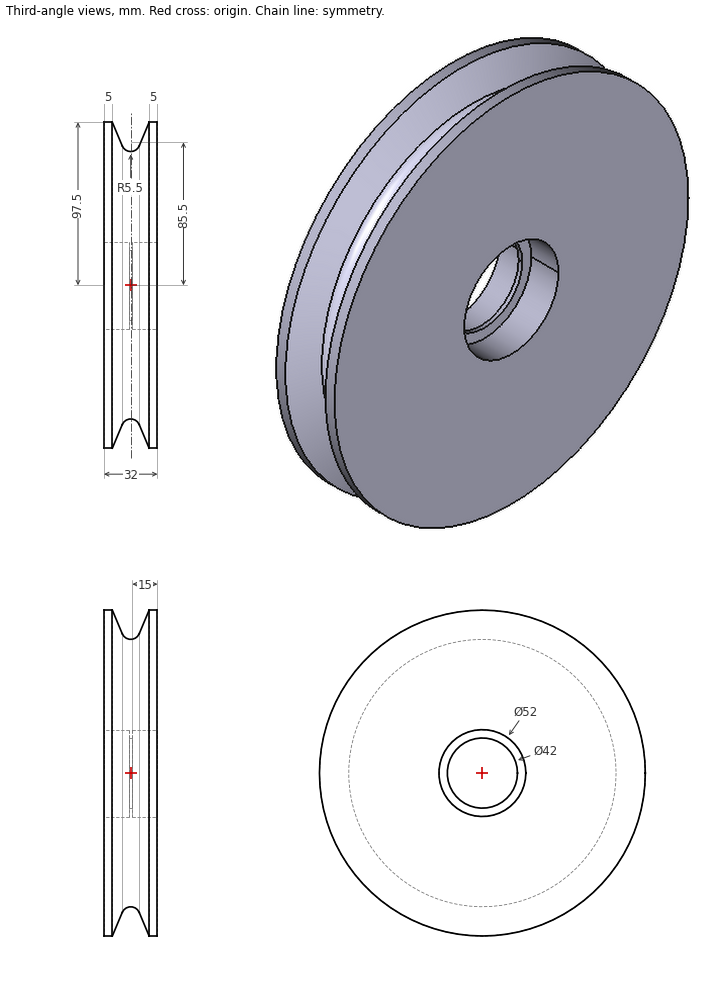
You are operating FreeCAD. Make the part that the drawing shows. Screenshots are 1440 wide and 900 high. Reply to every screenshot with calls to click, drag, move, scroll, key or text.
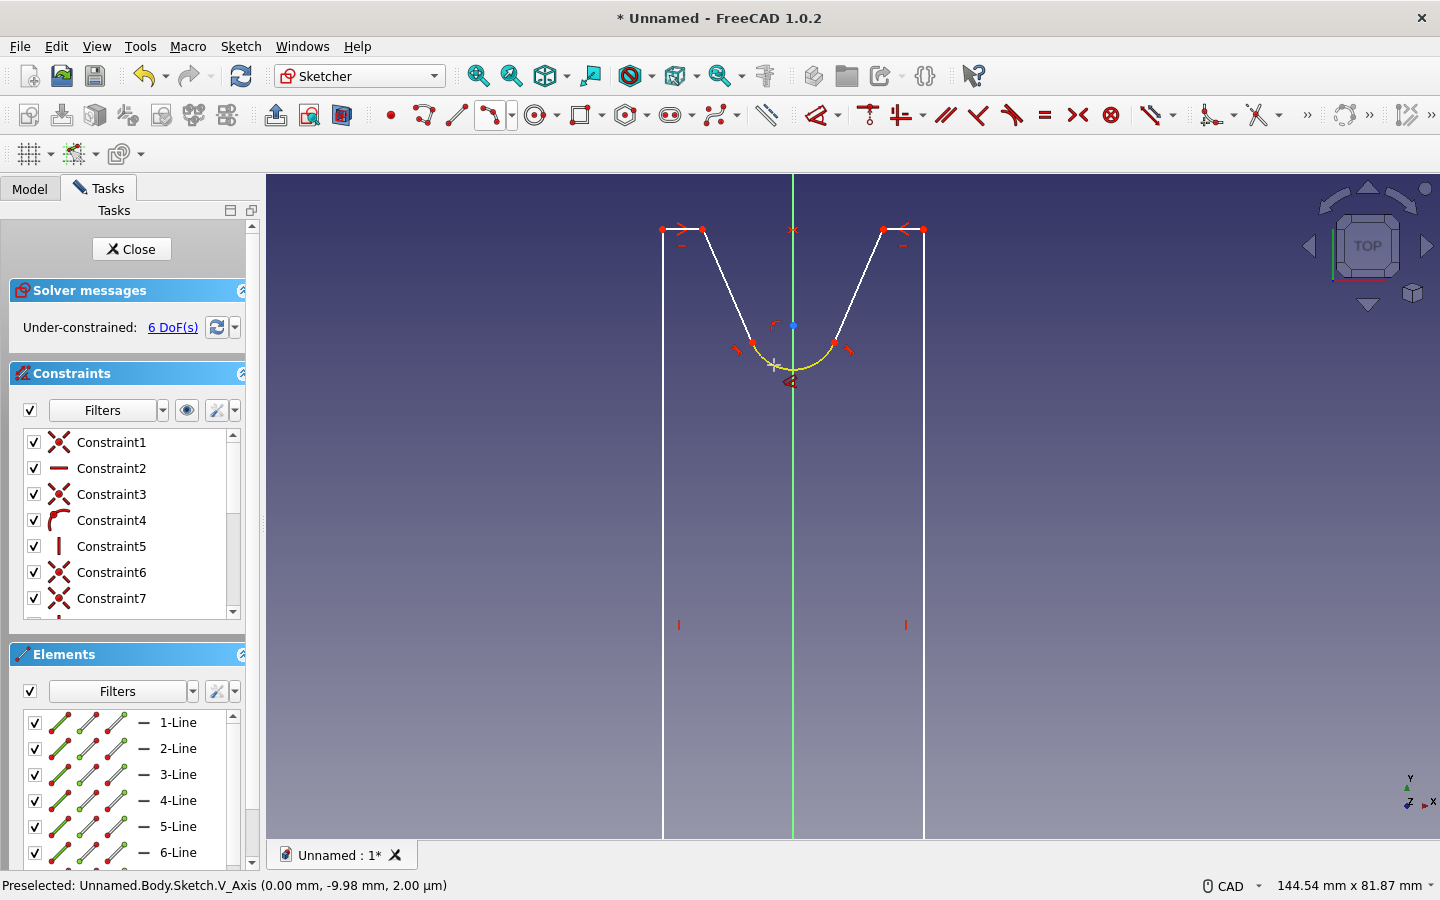
click(773, 365)
click(759, 394)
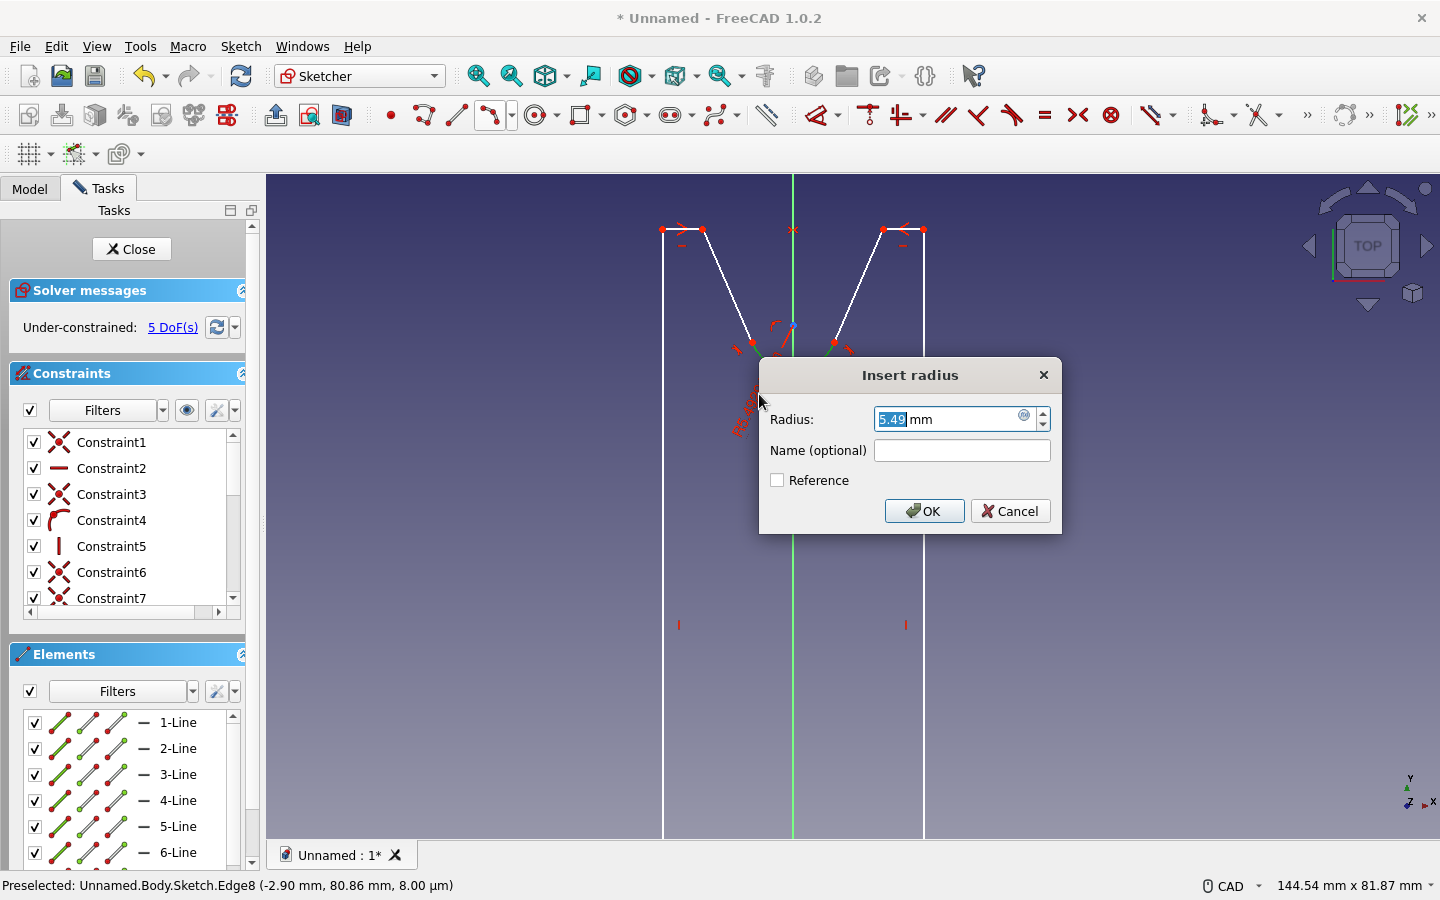
text(5.5)
key(Return)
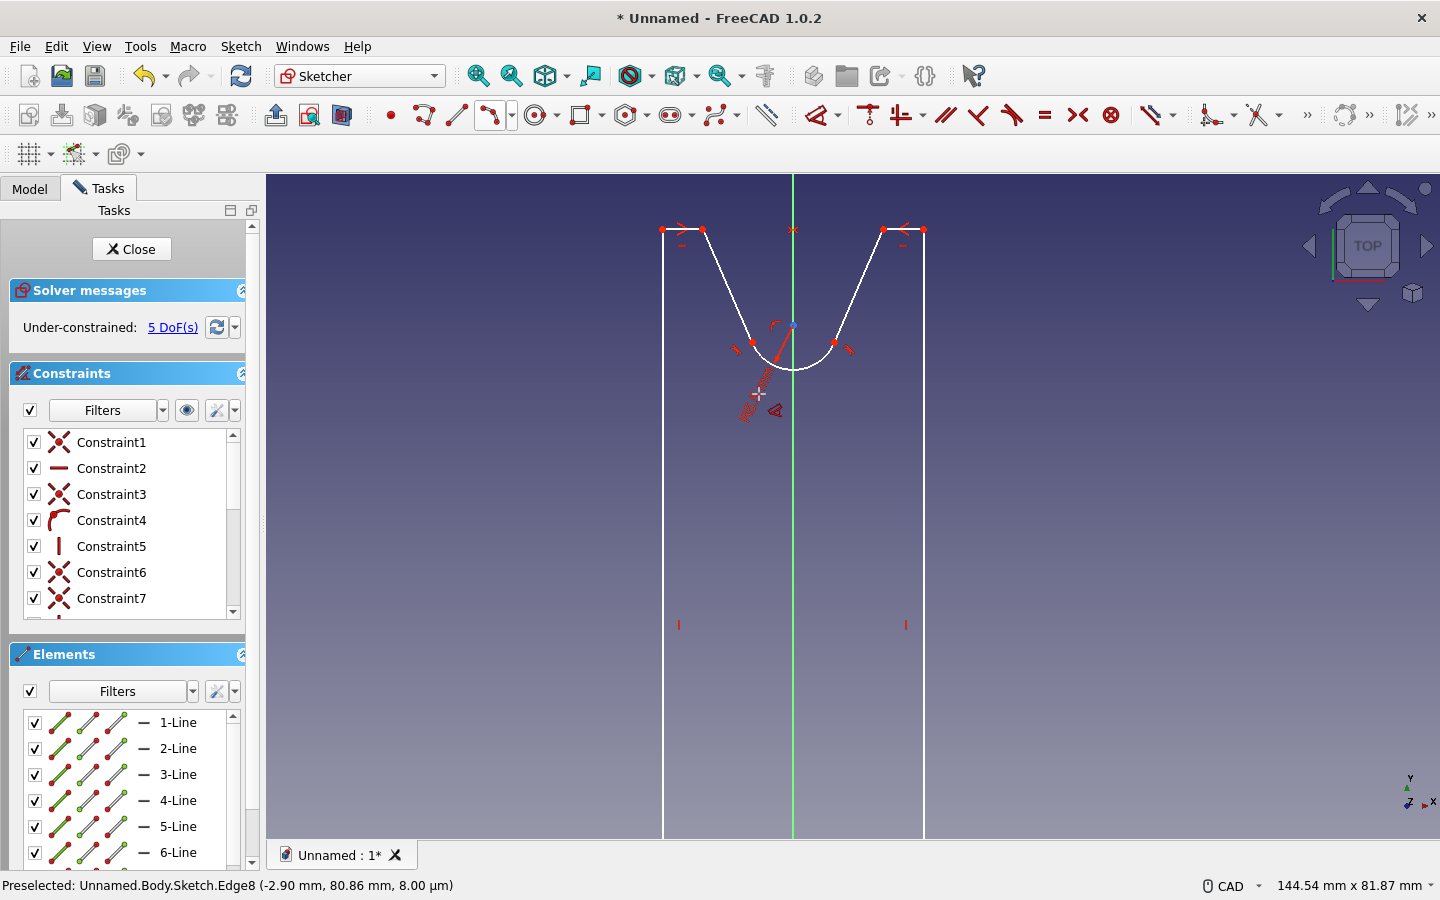
click(691, 229)
click(683, 263)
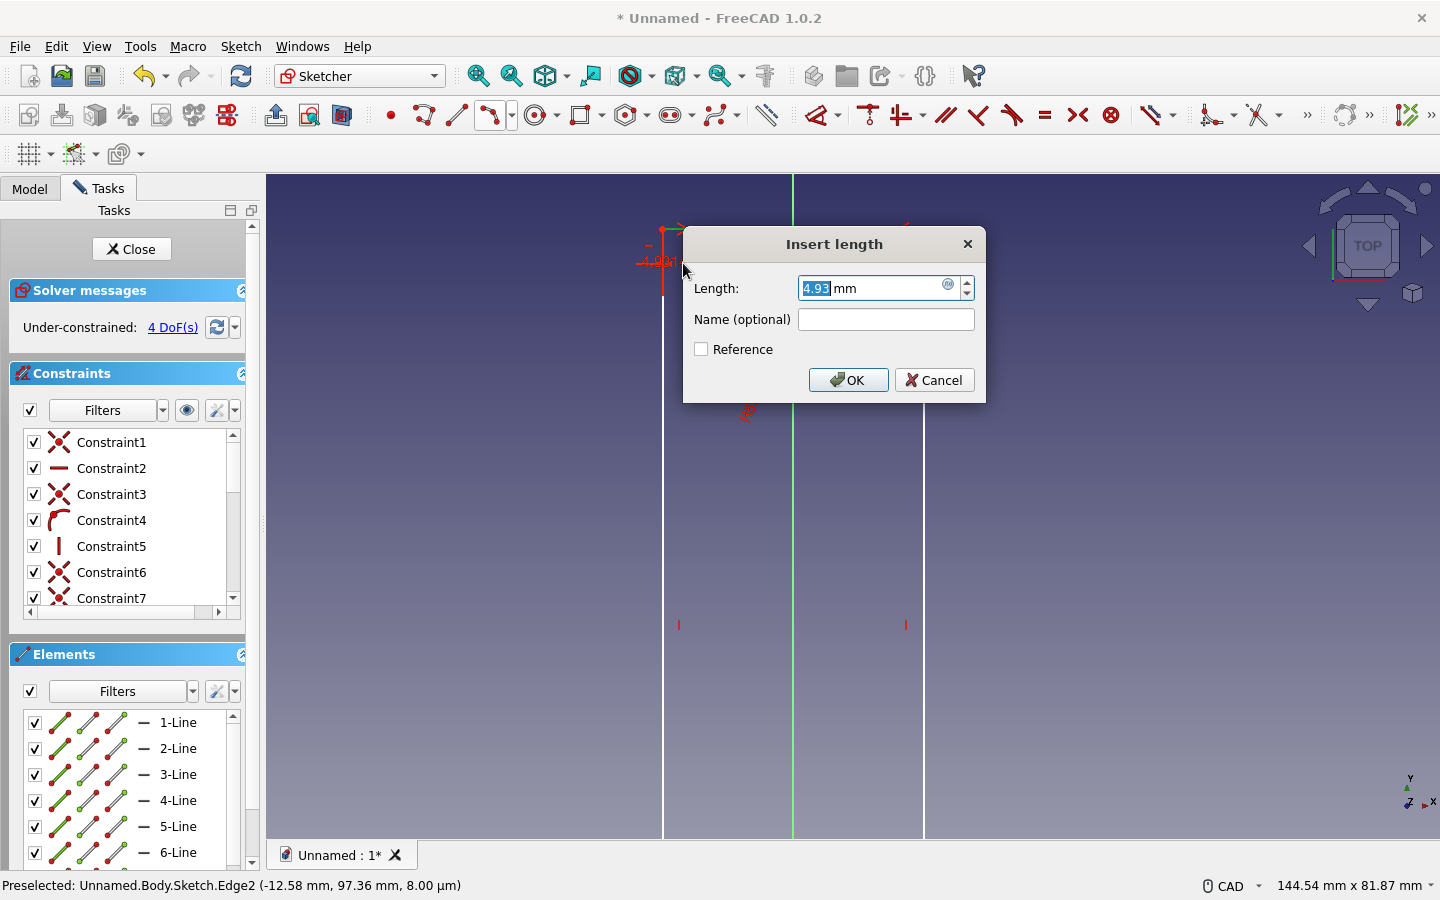
text(5)
key(Return)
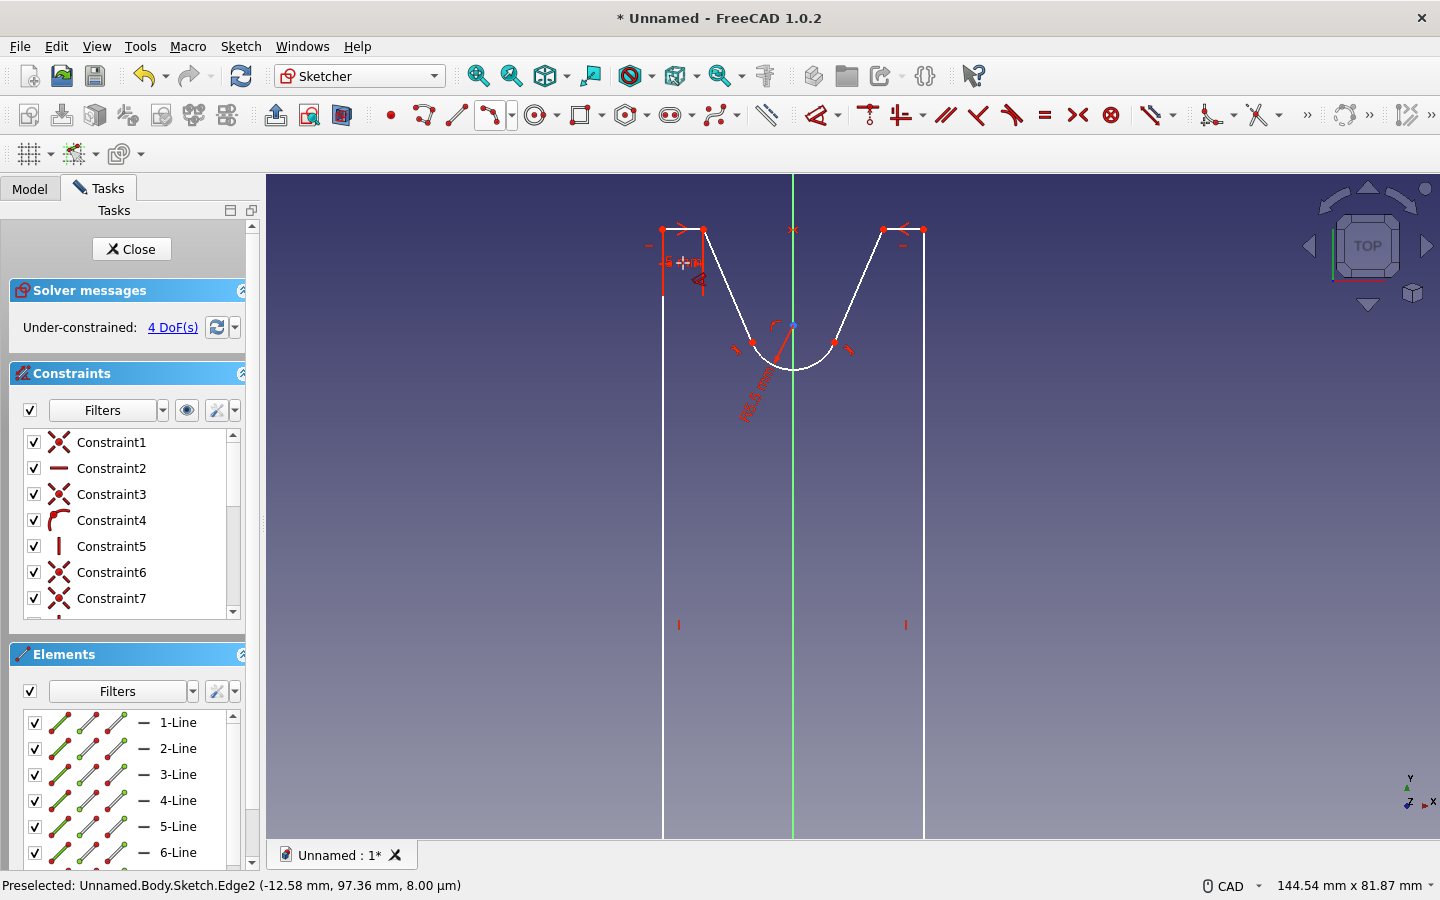
click(911, 229)
click(903, 263)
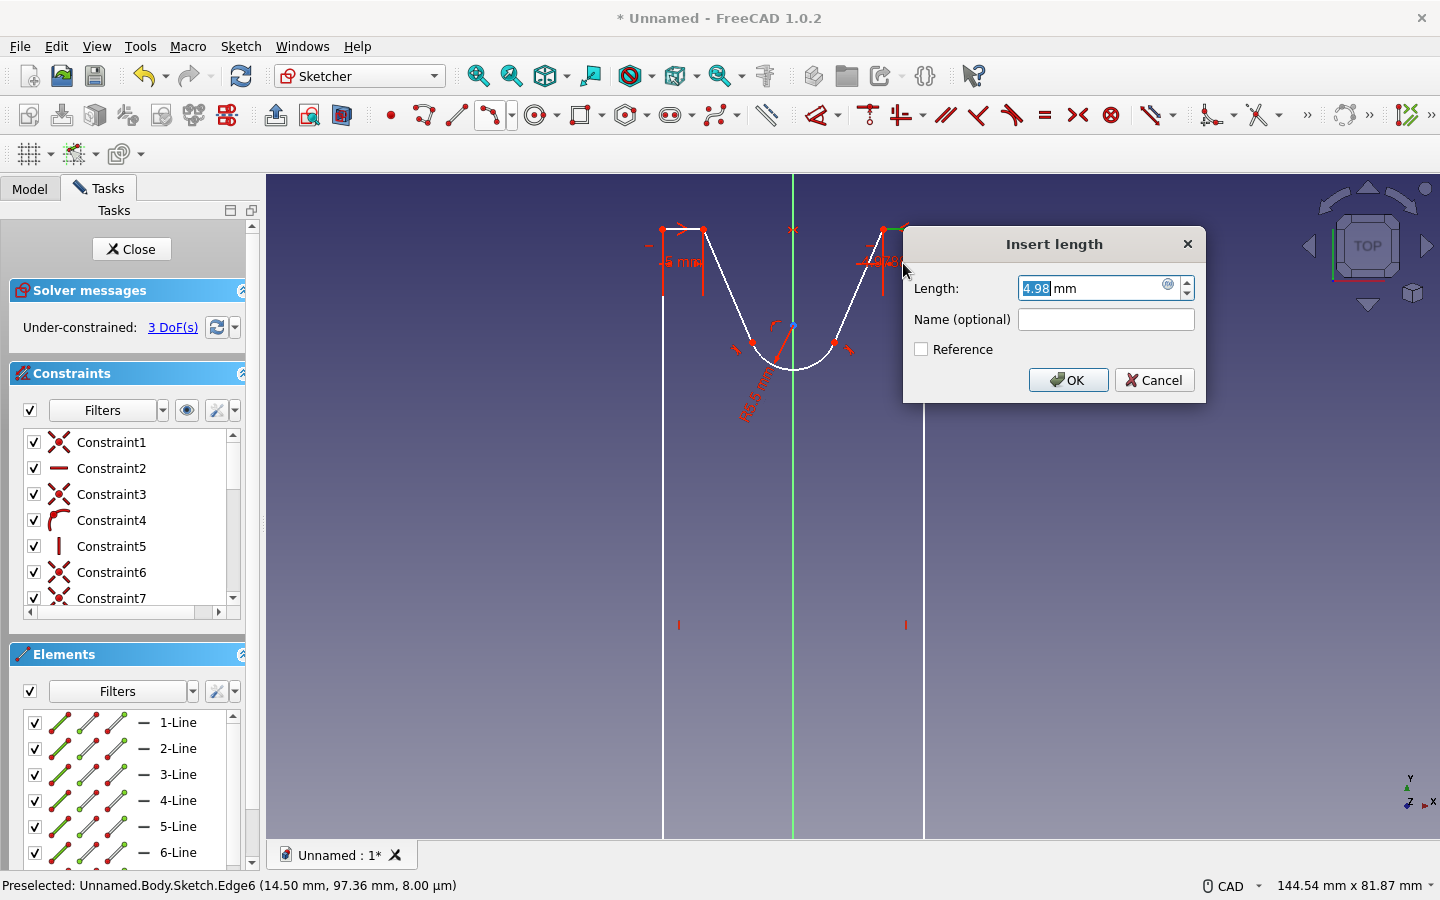
text(5)
key(Return)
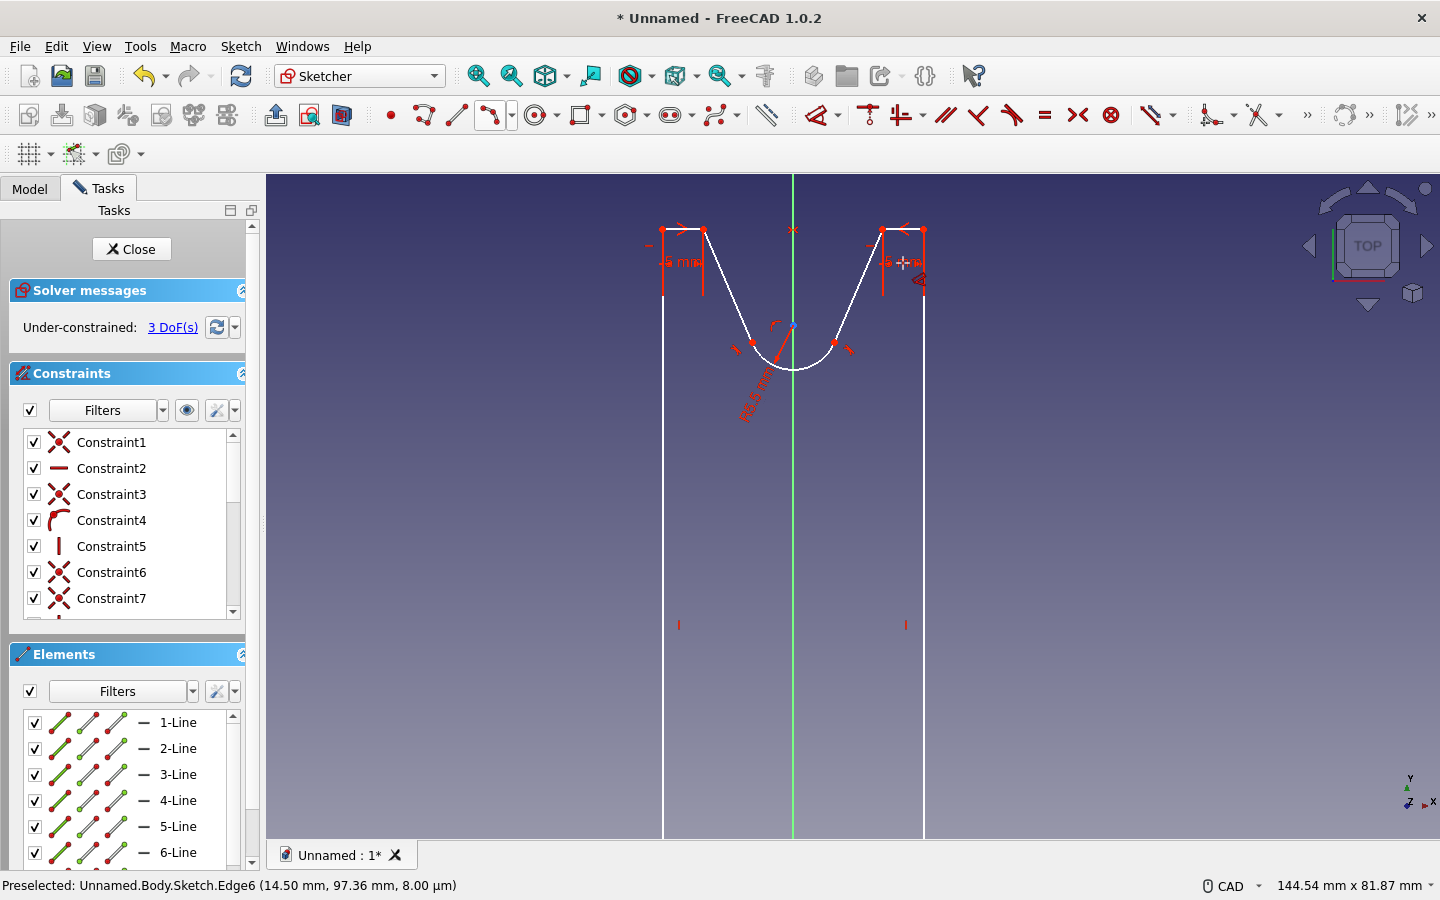
scroll(774, 364, down, 3)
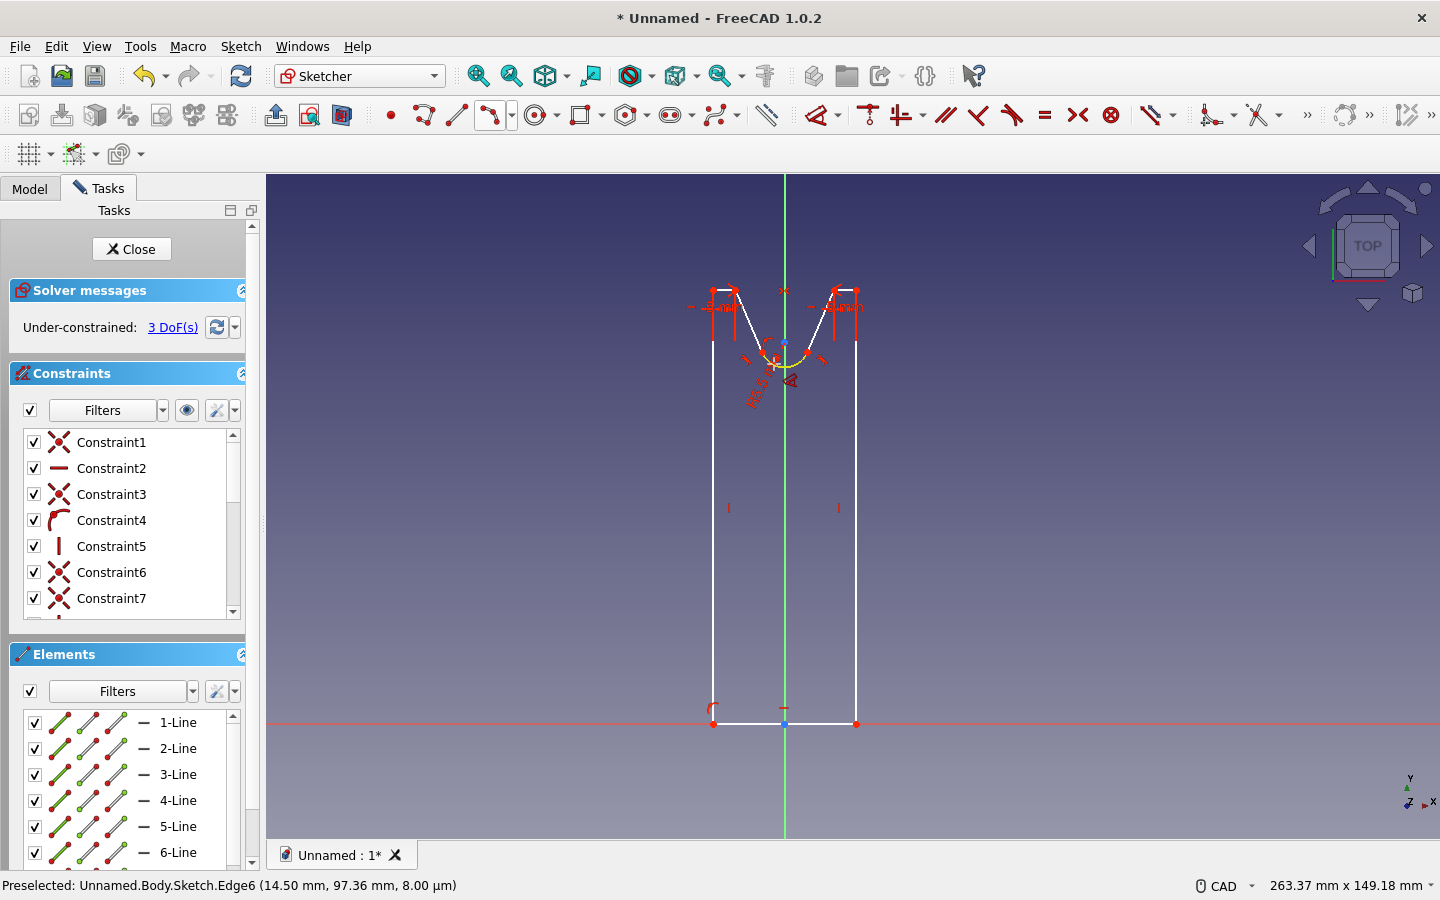
click(756, 724)
click(752, 758)